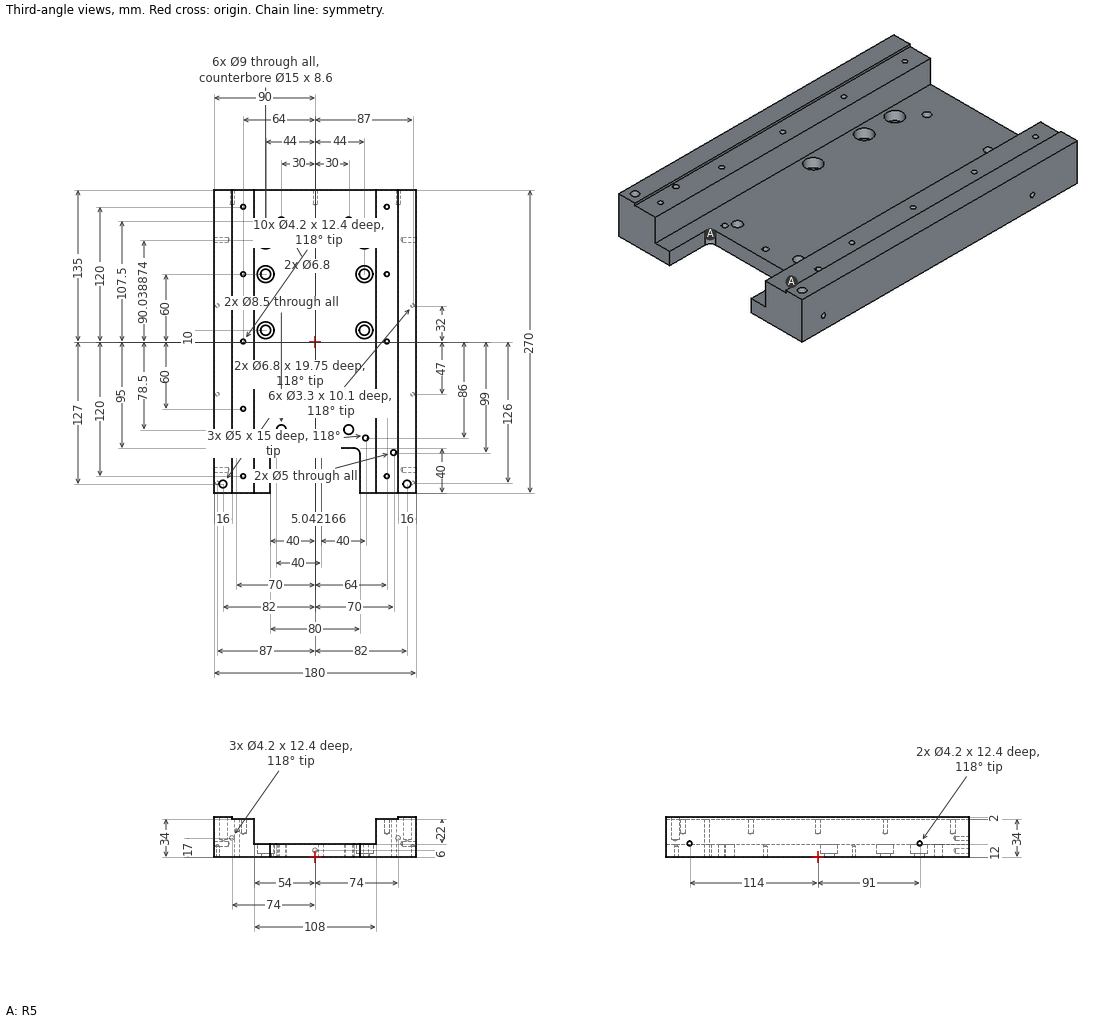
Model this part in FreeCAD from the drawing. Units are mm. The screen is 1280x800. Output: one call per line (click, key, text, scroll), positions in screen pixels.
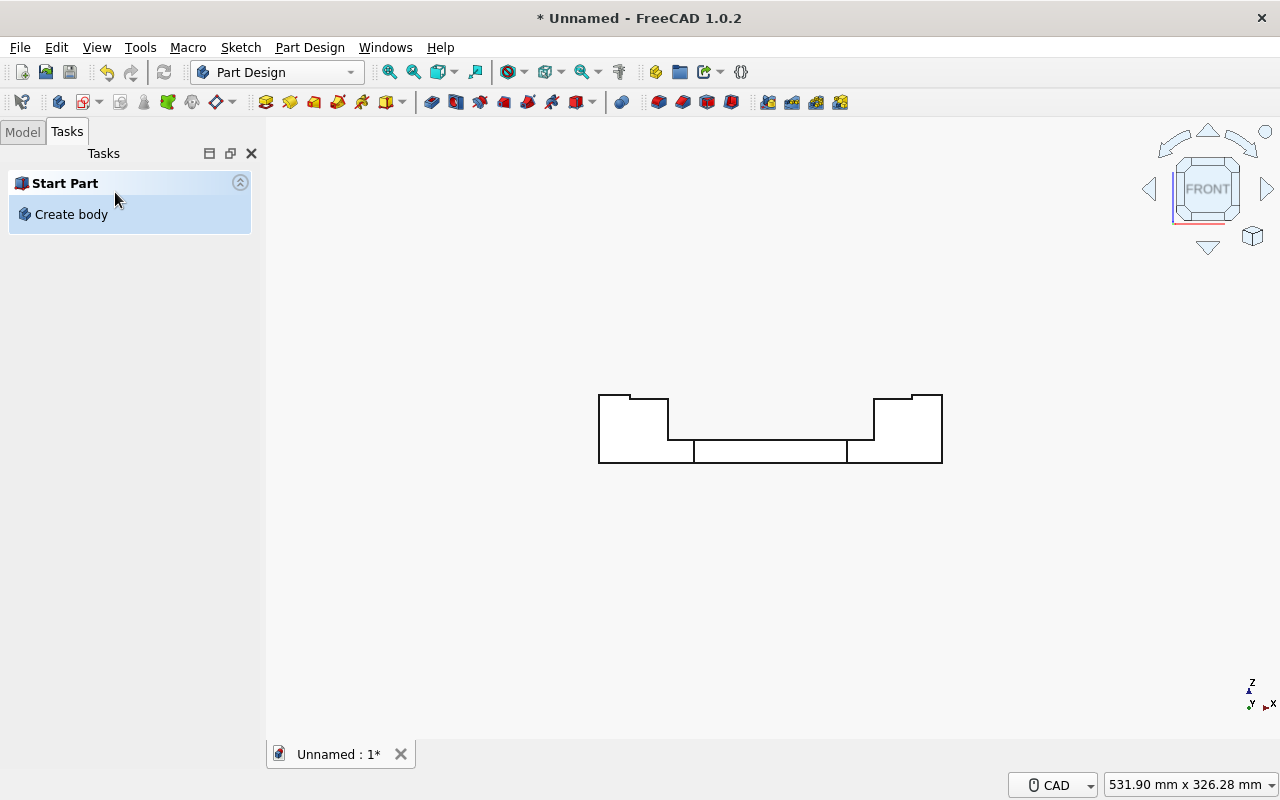
key(v)
key(f)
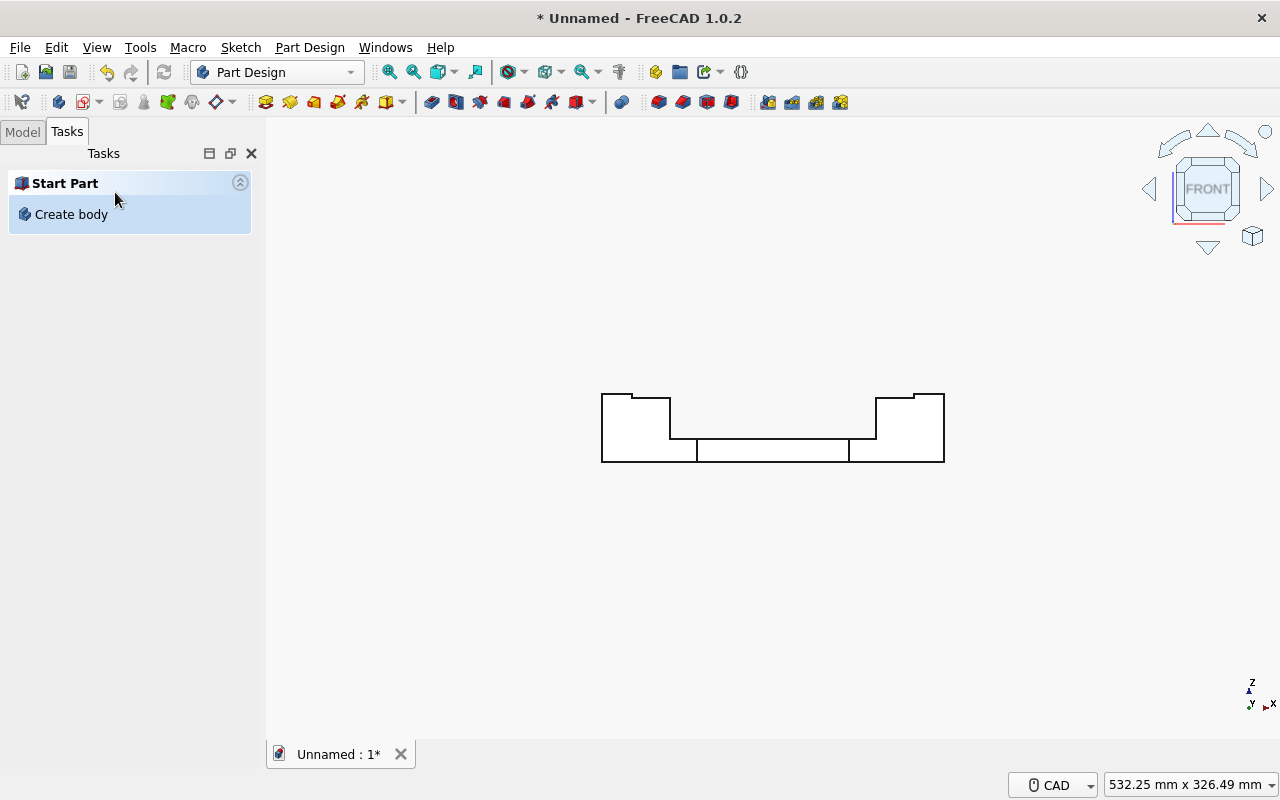
key(3)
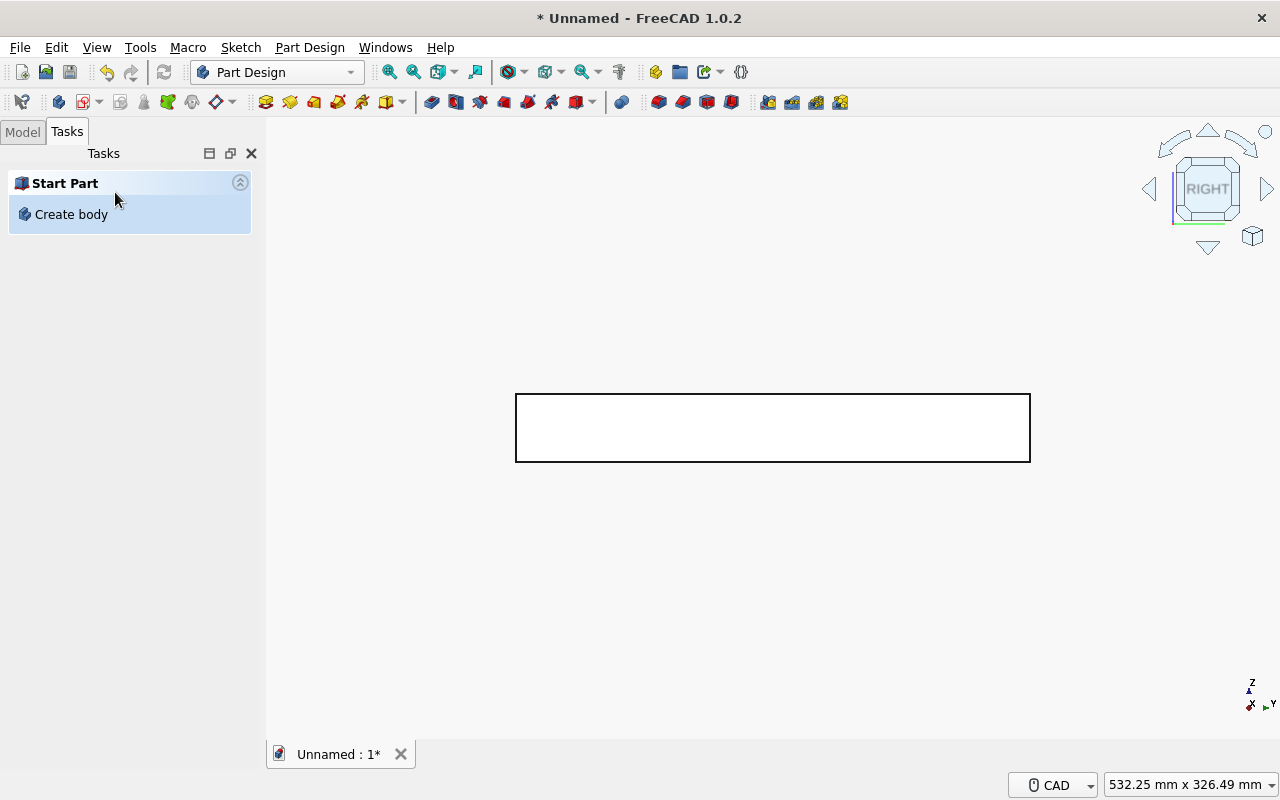
key(5)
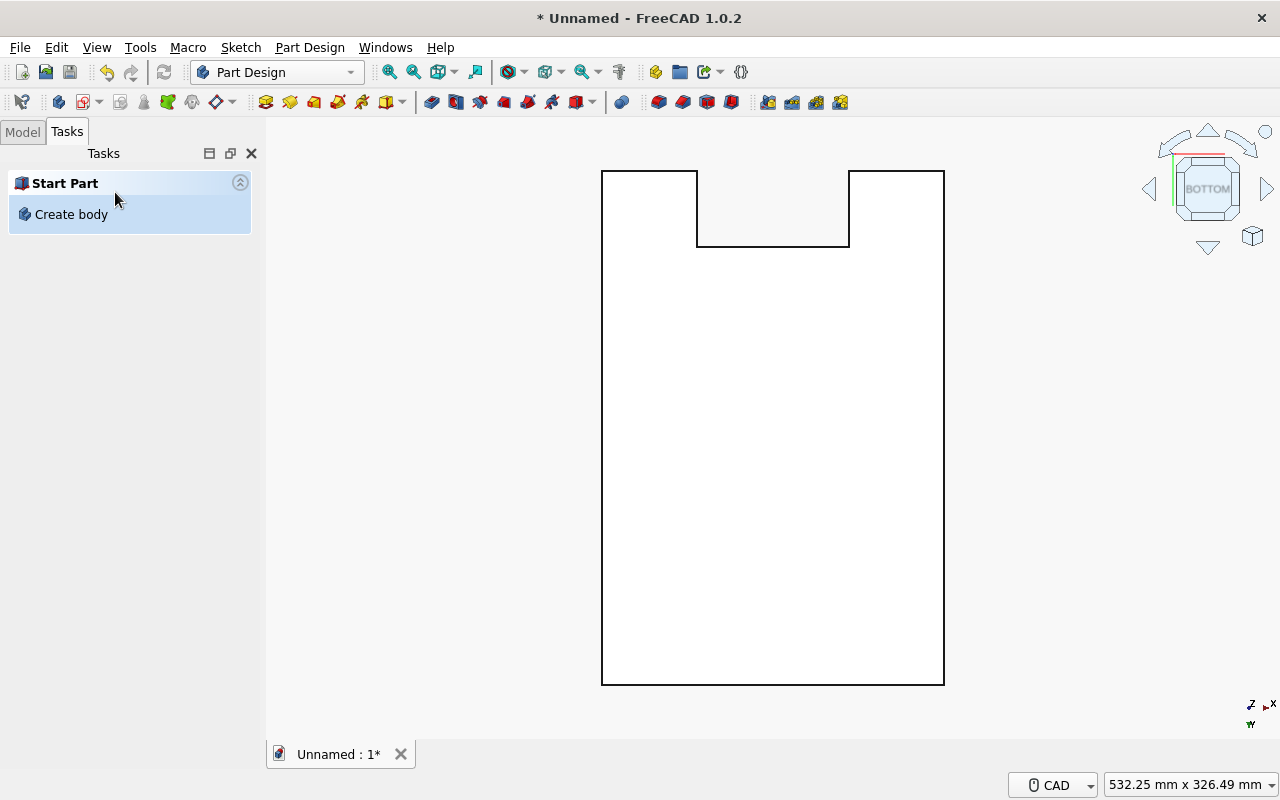
key(4)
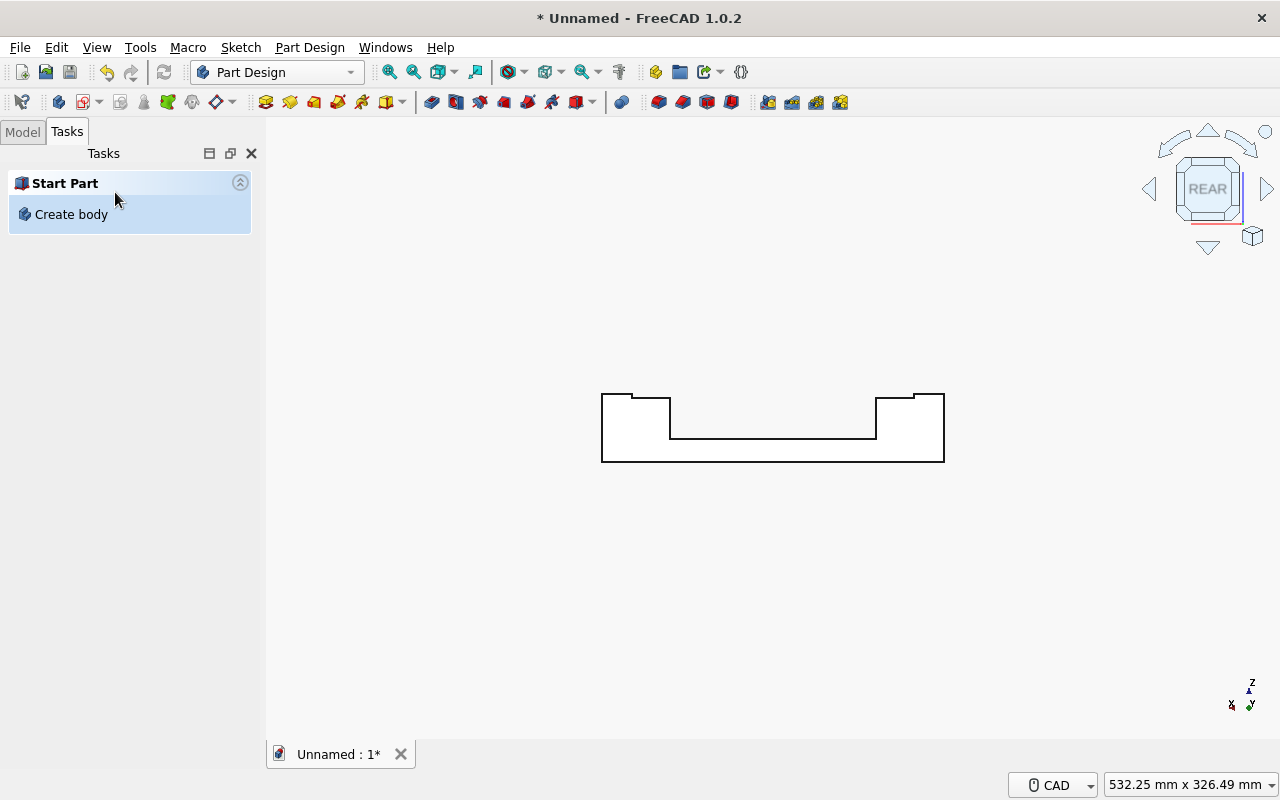
click(390, 72)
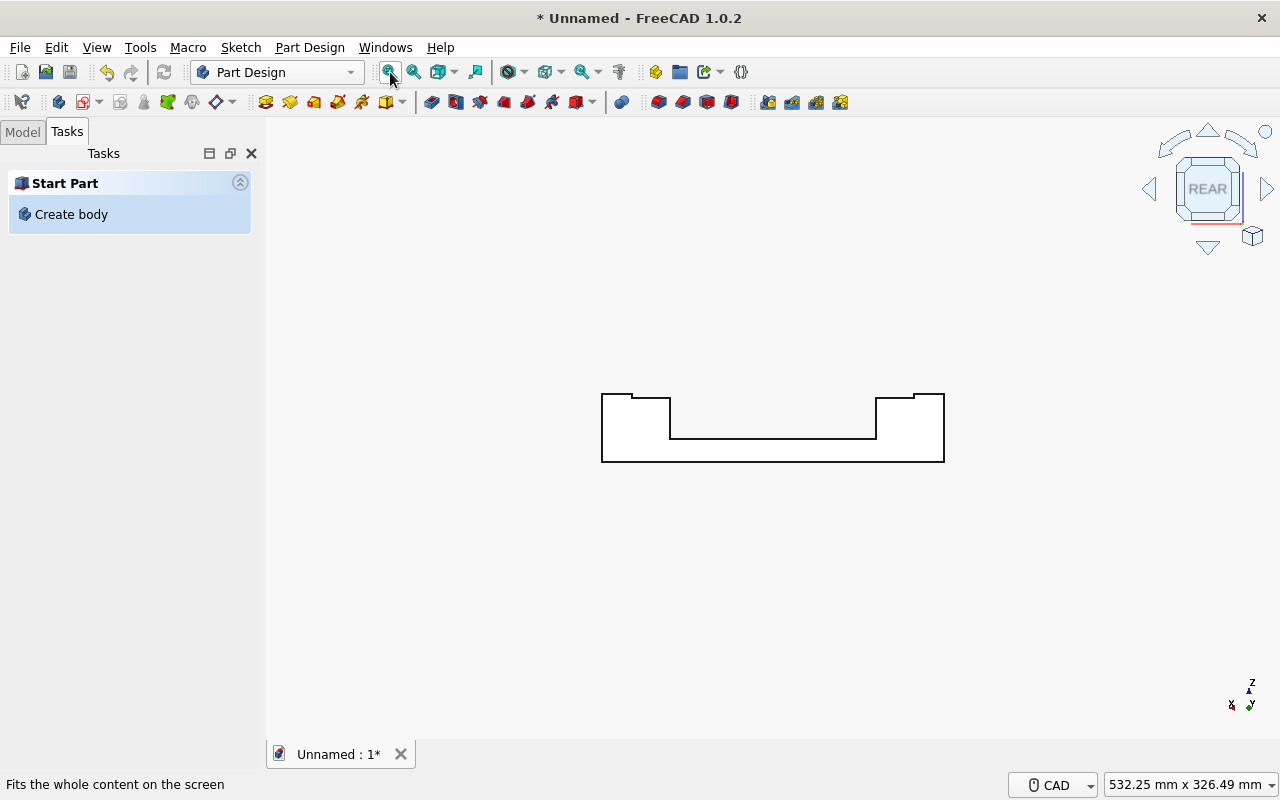
key(6)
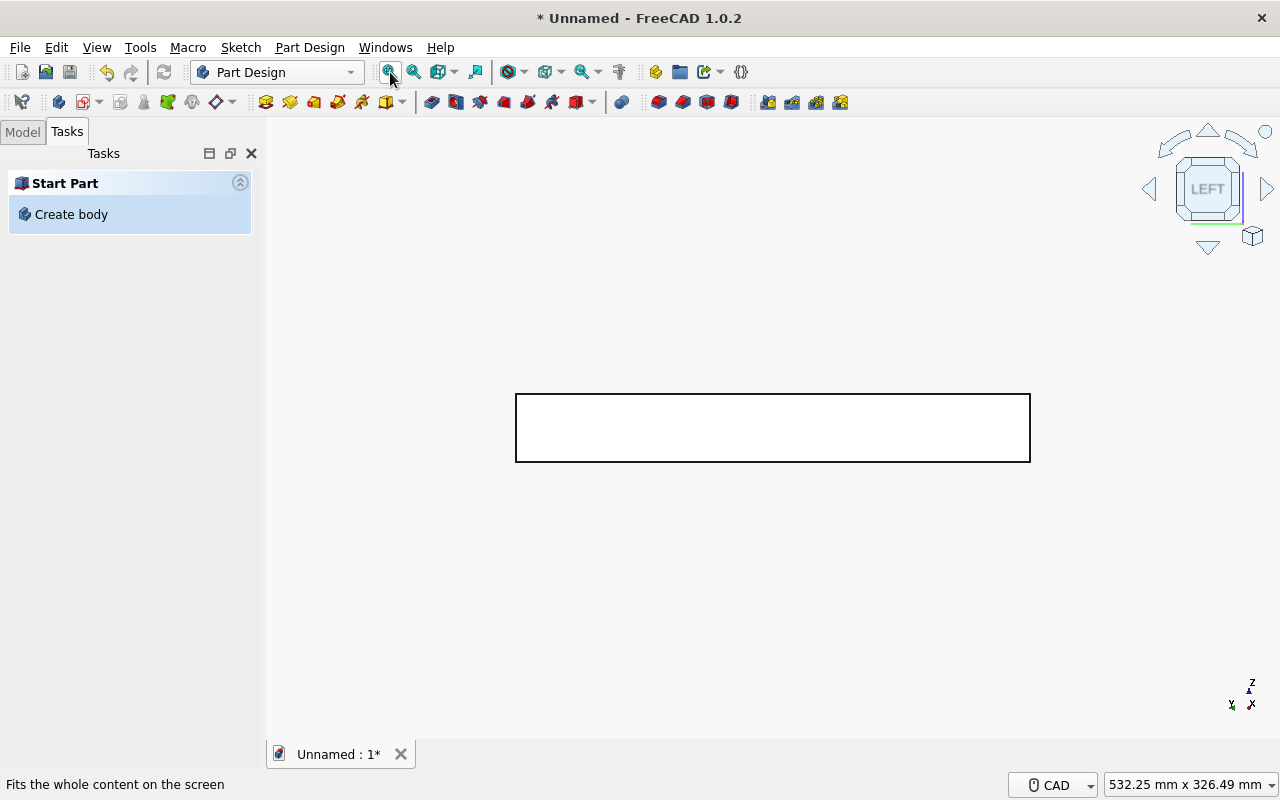
key(v)
key(3)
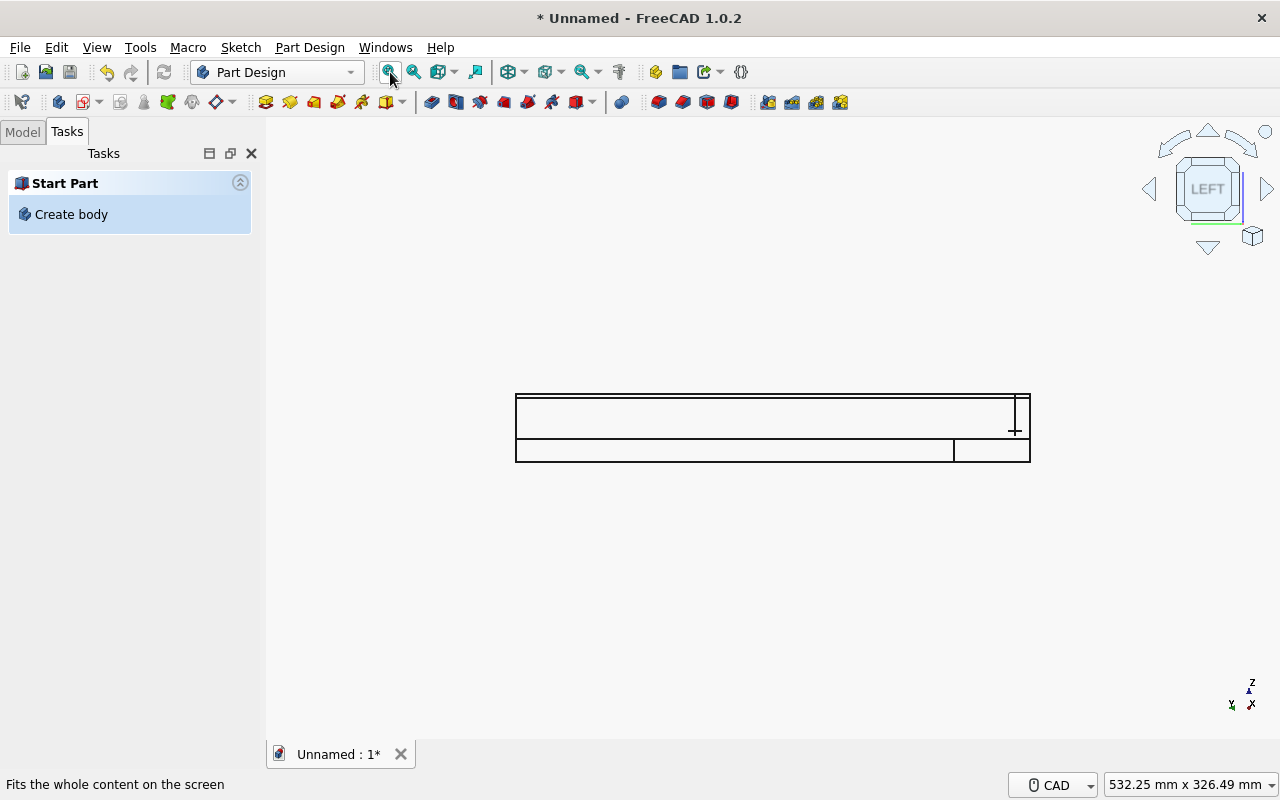
key(0)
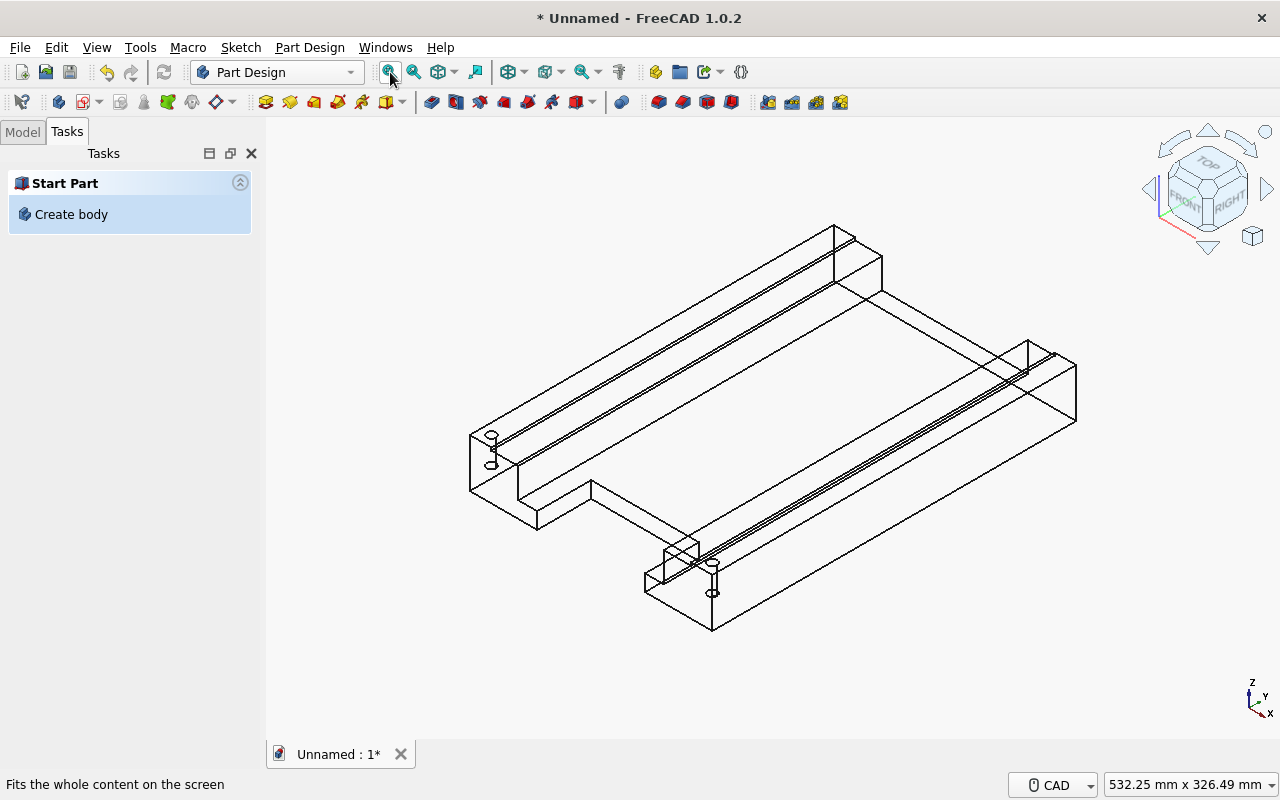
click(699, 549)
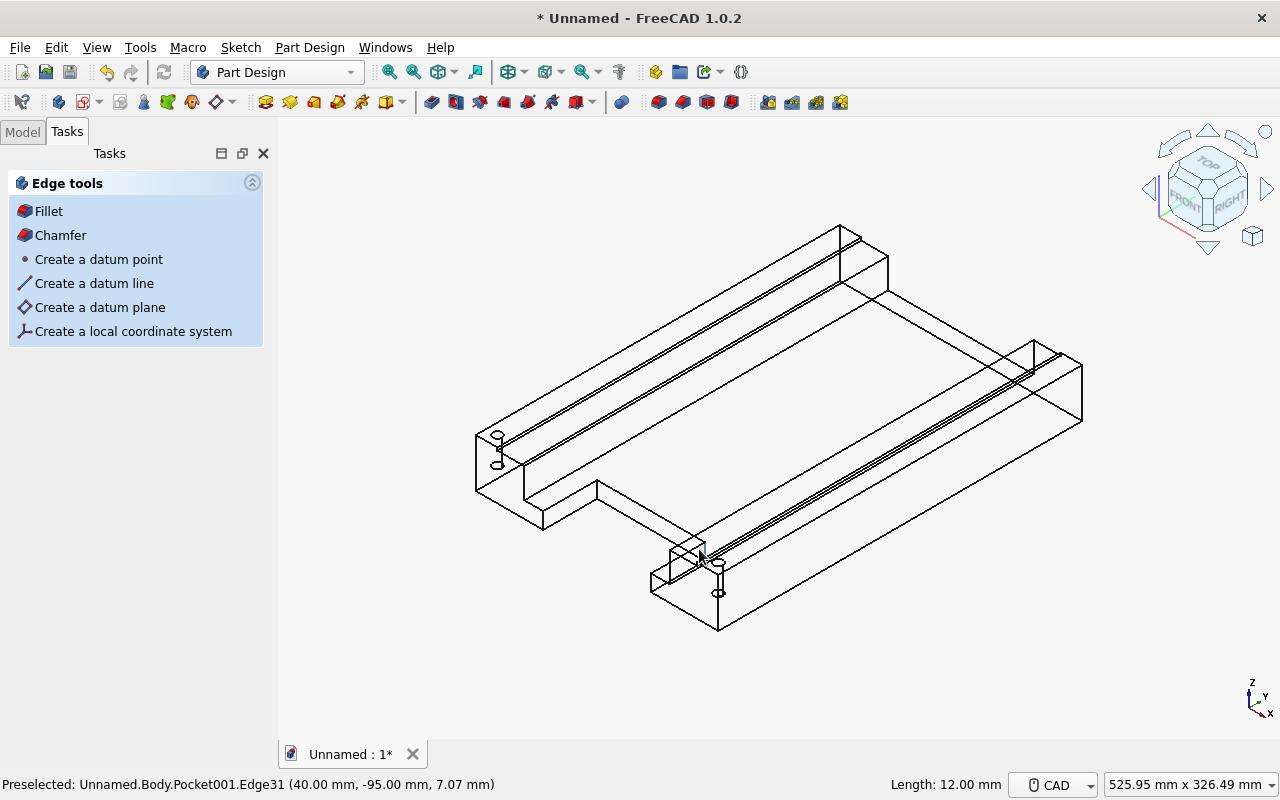
click(597, 488, ctrl)